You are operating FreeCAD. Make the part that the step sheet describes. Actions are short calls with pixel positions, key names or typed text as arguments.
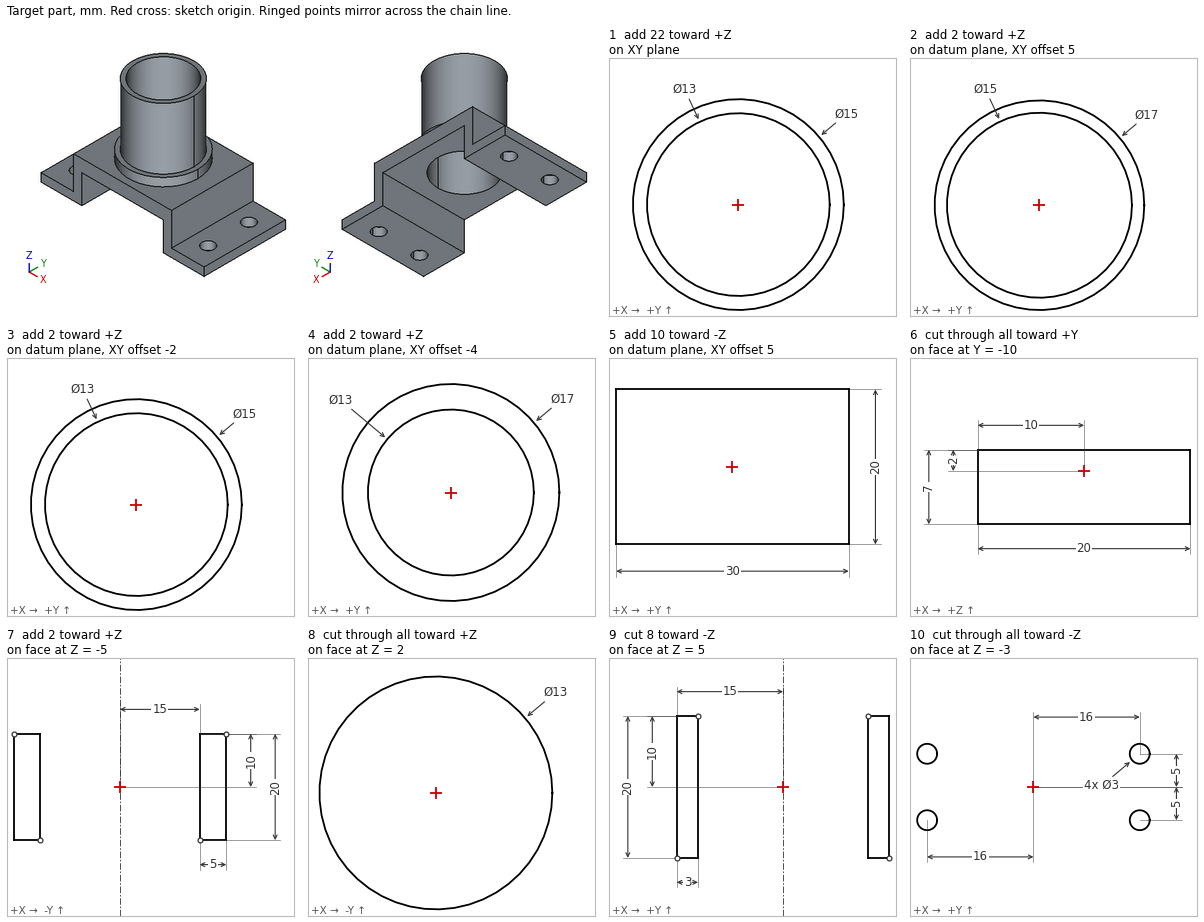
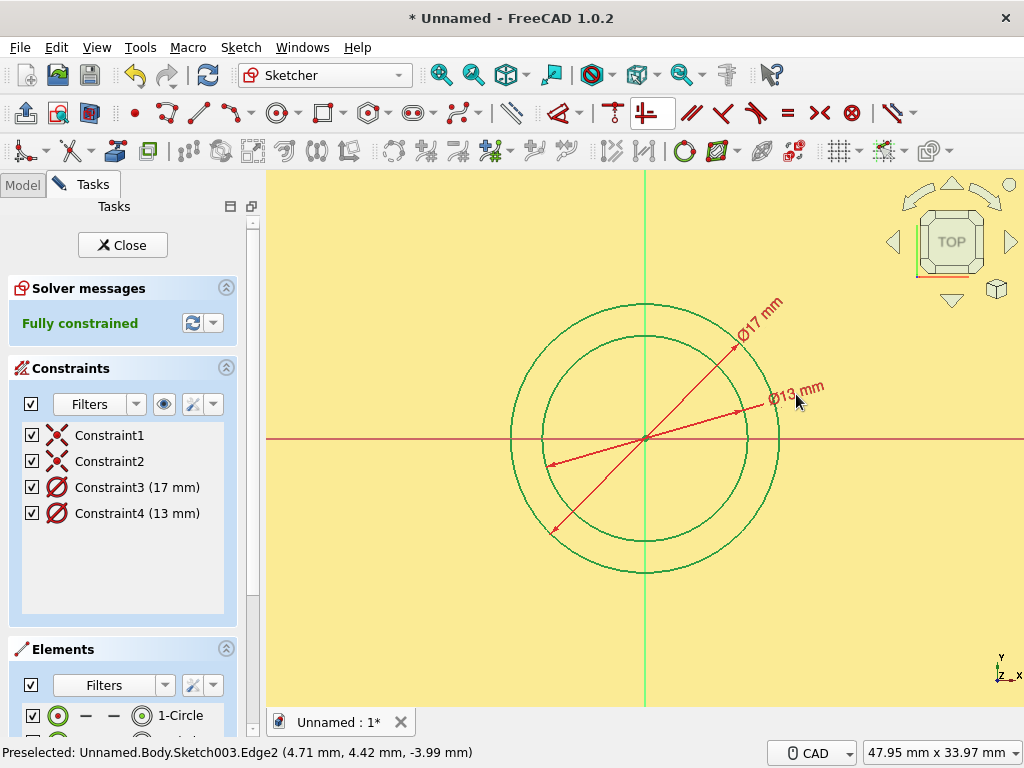
click(123, 245)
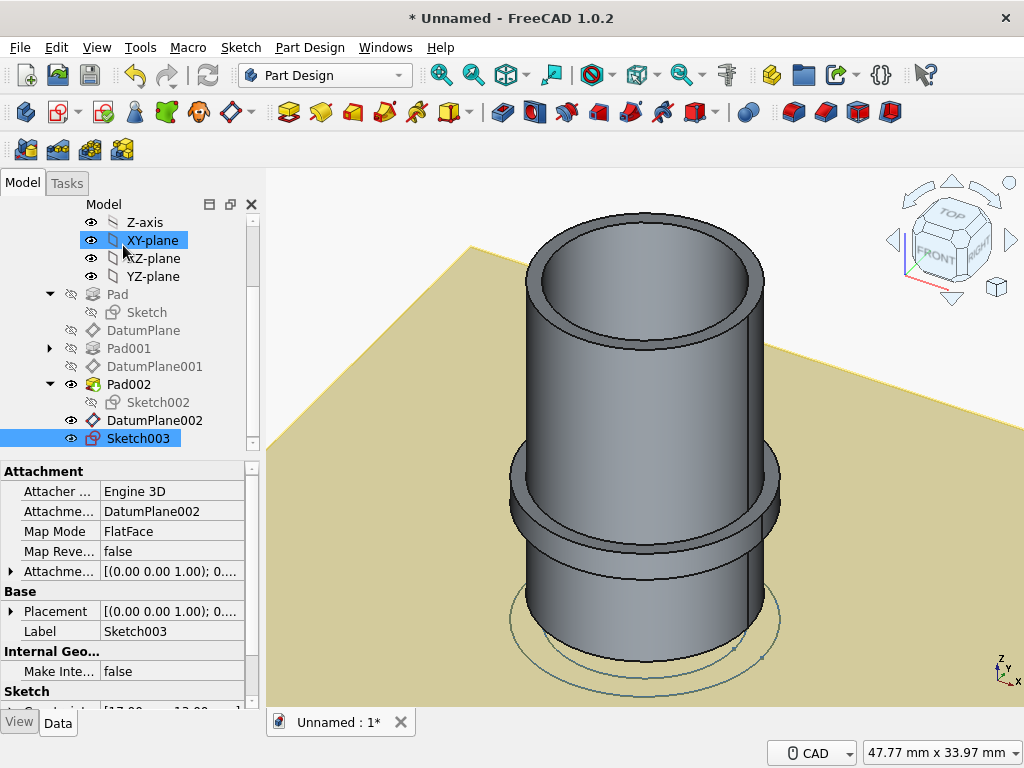
click(290, 112)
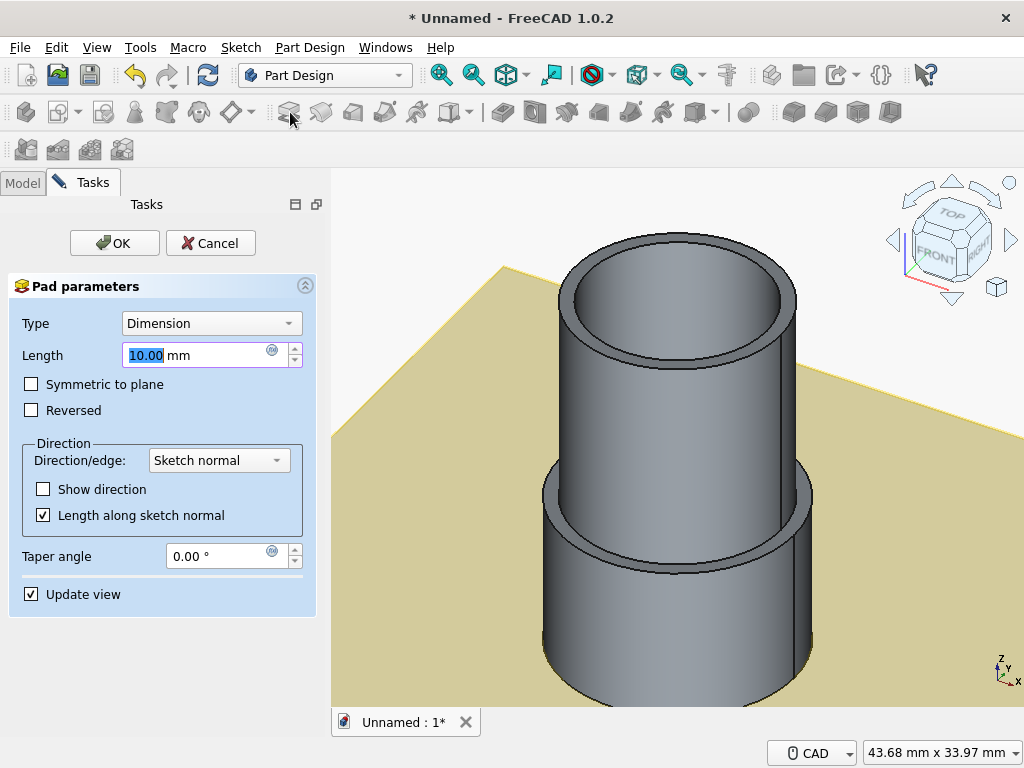
text(2)
key(Tab)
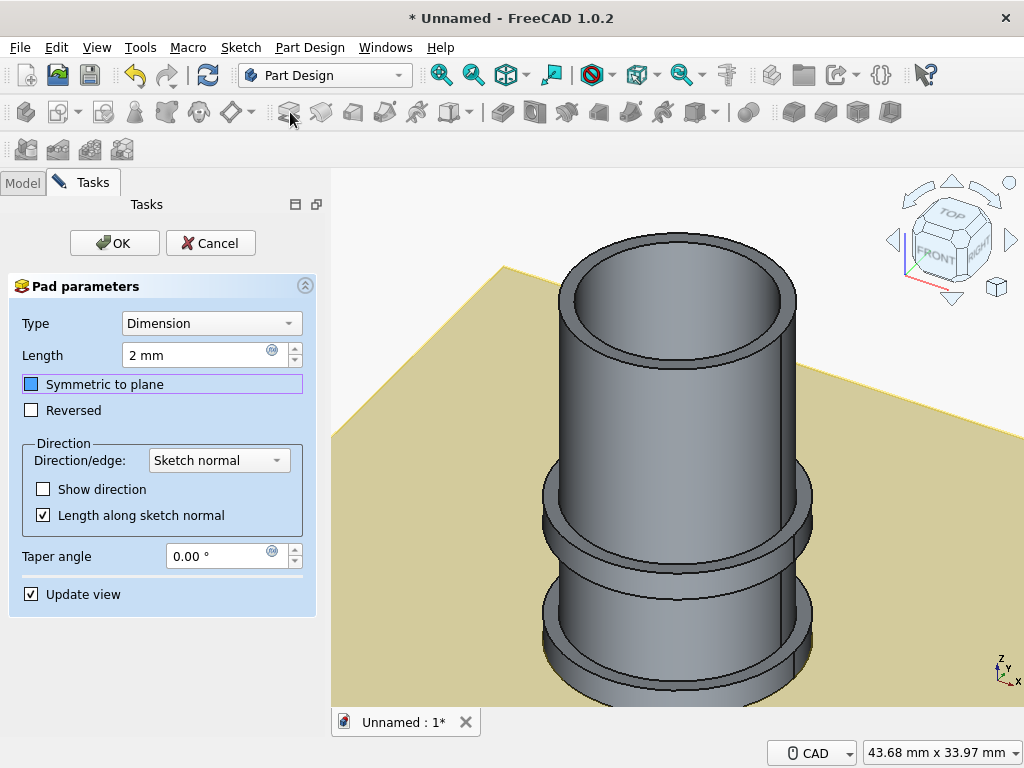
click(115, 243)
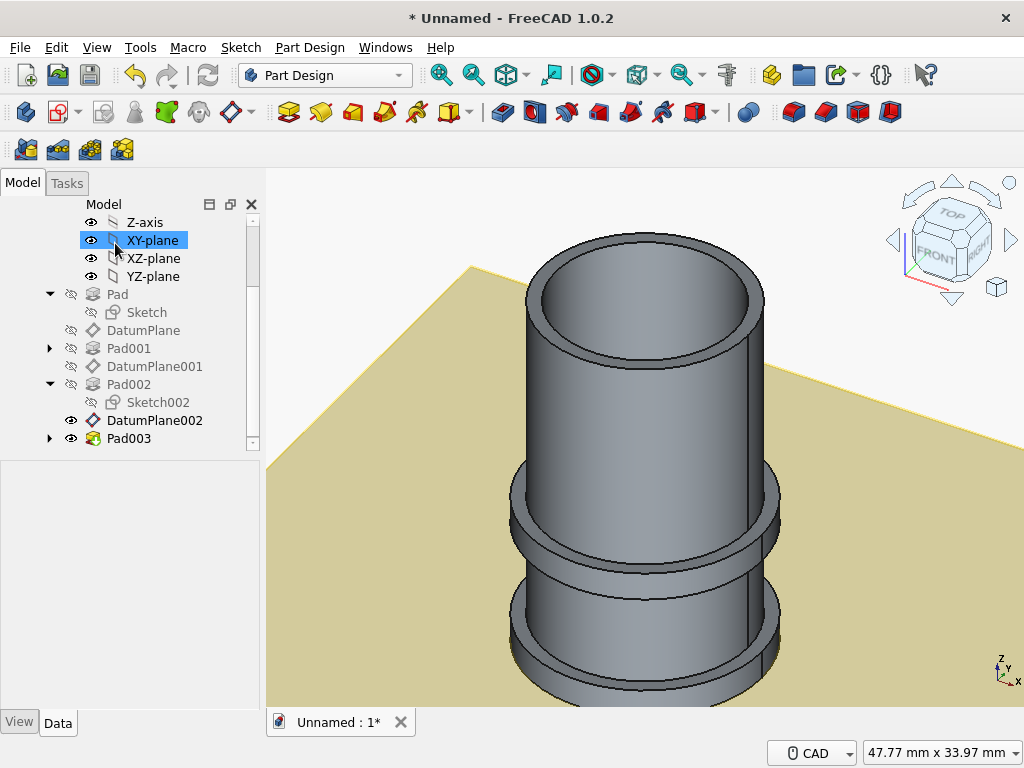
click(116, 420)
key(space)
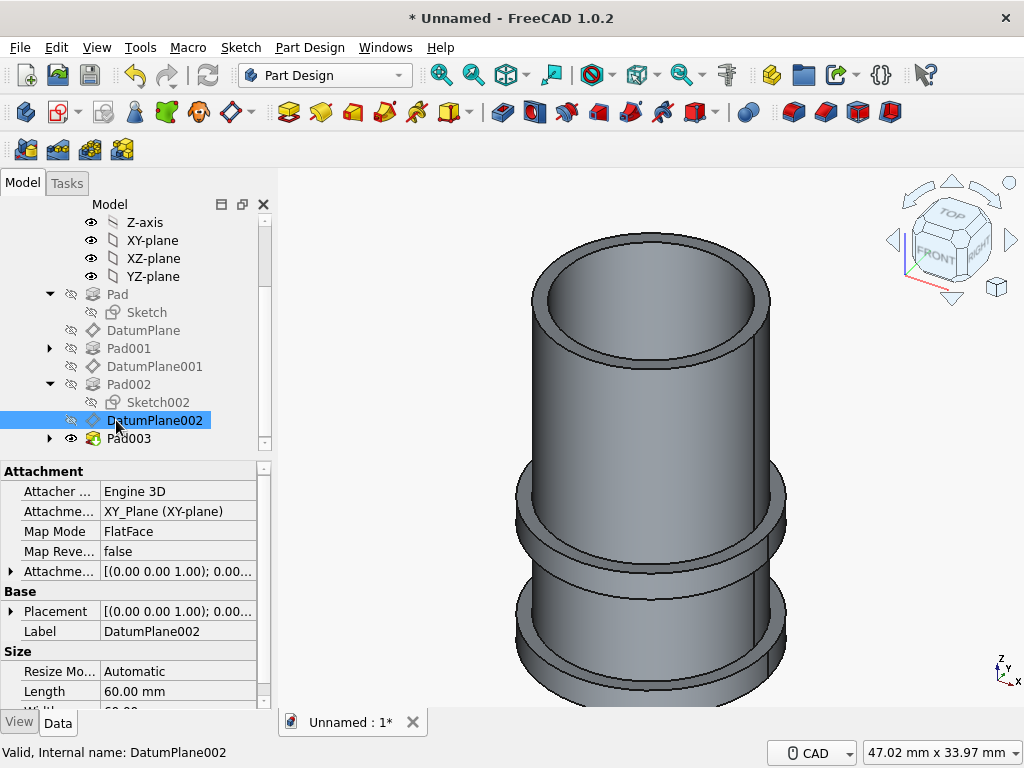
click(442, 76)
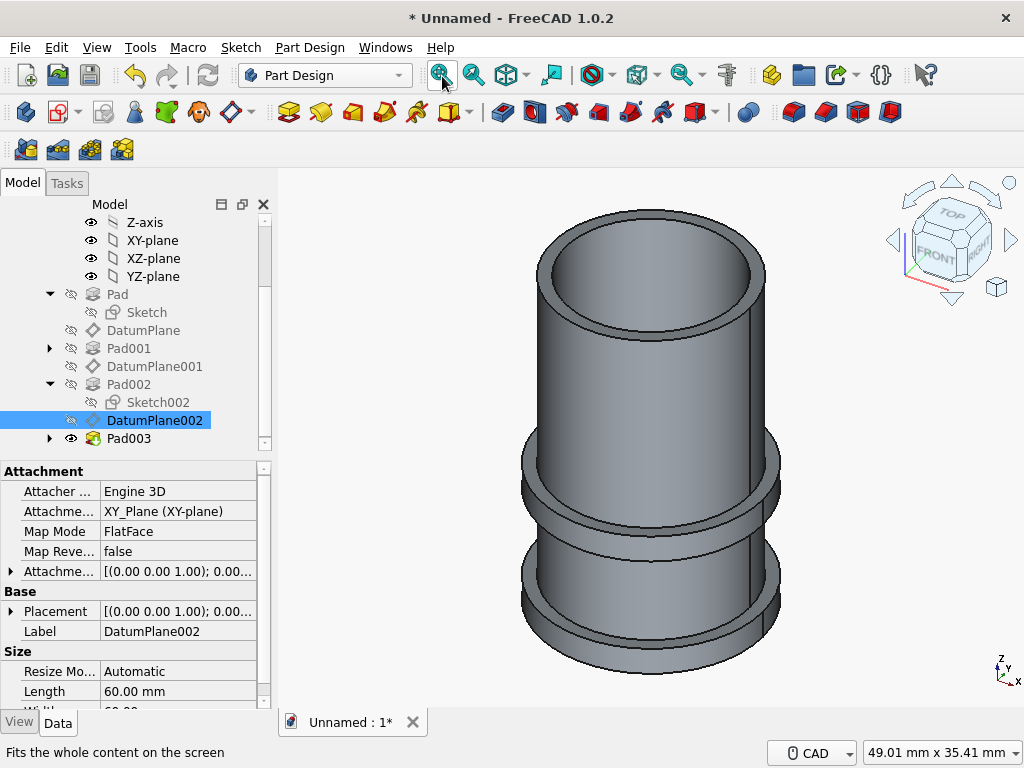
scroll(160, 326, down, 3)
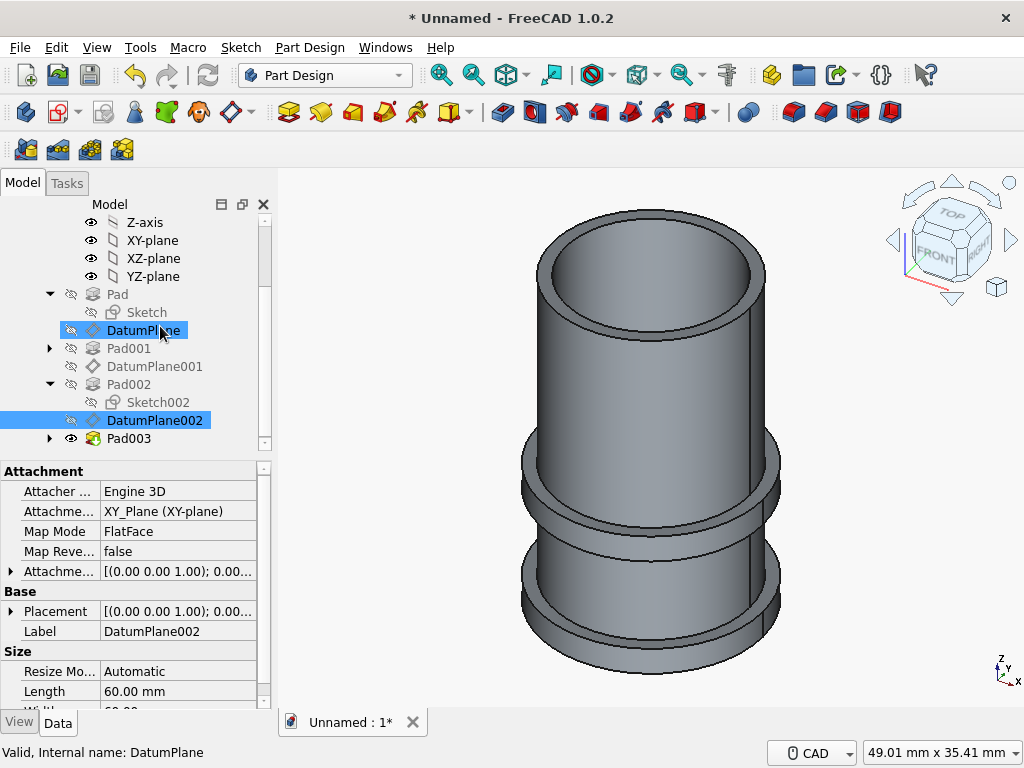
scroll(160, 326, up, 15)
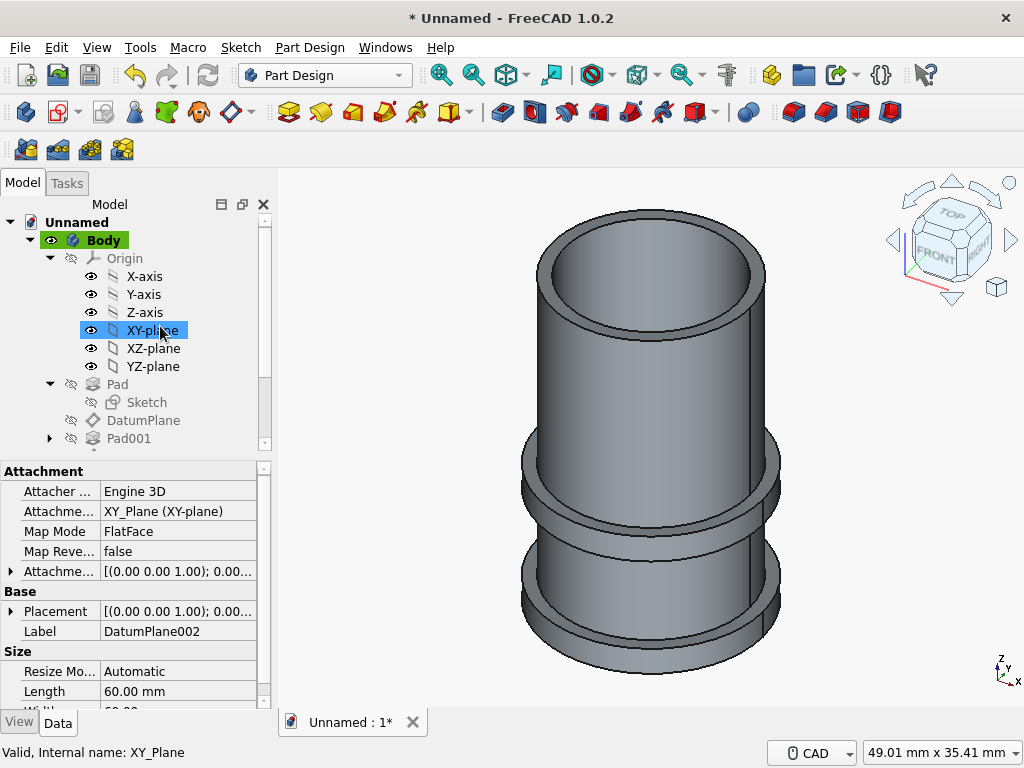
click(136, 330)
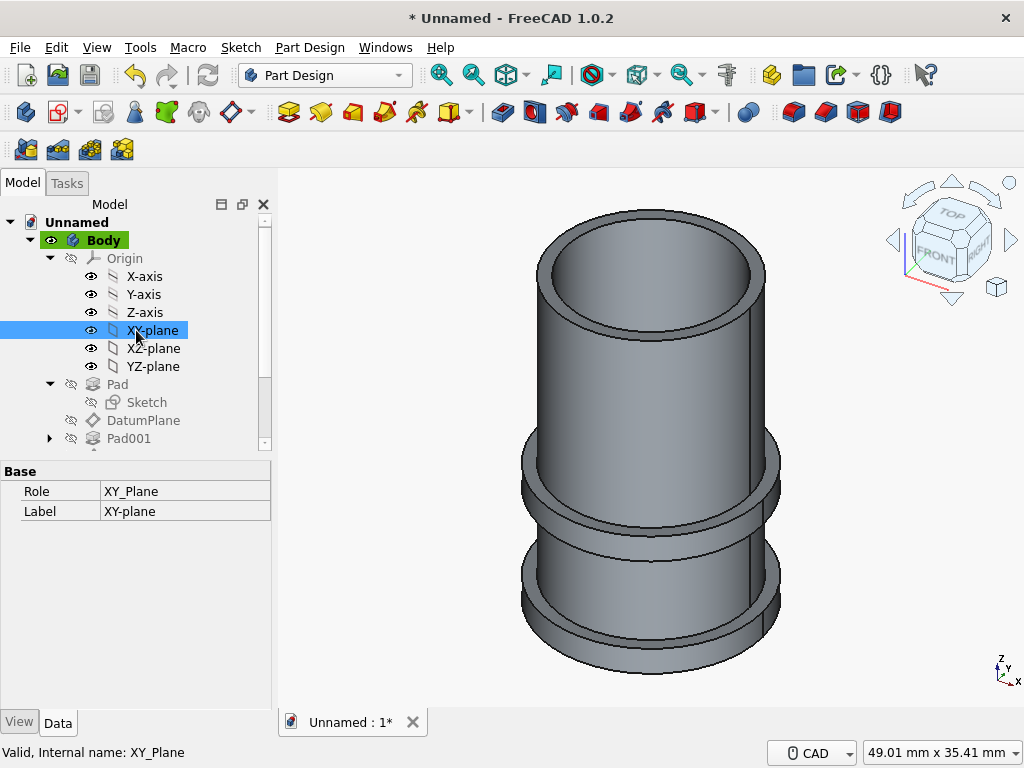
click(232, 112)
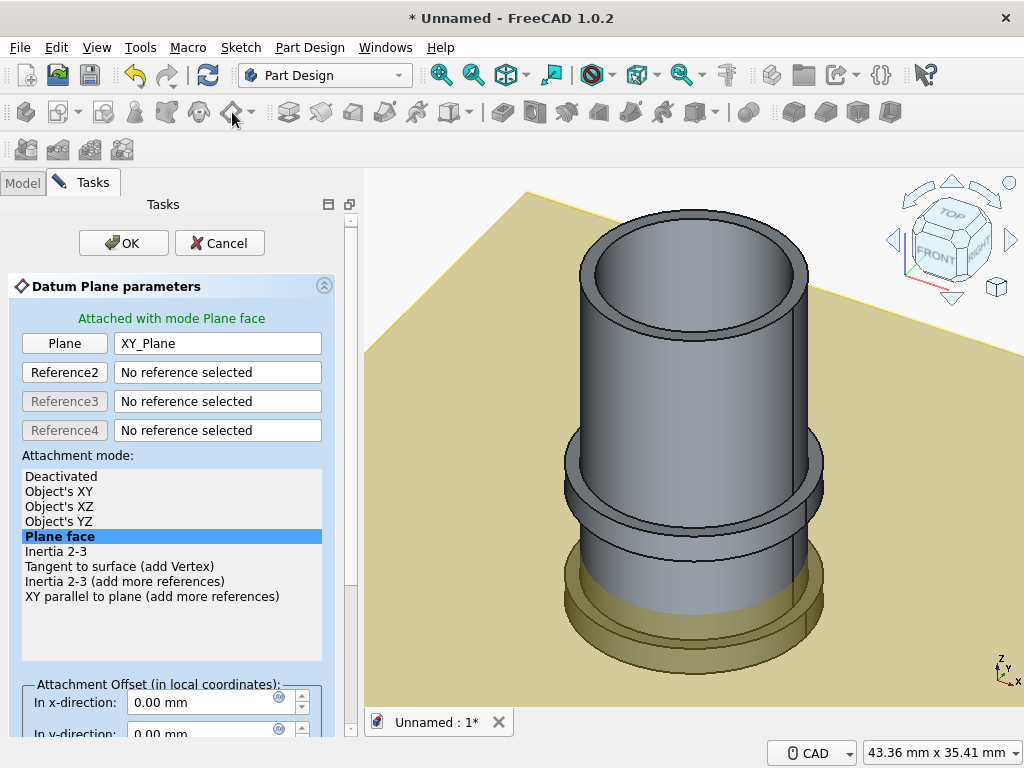
scroll(351, 475, down, 2)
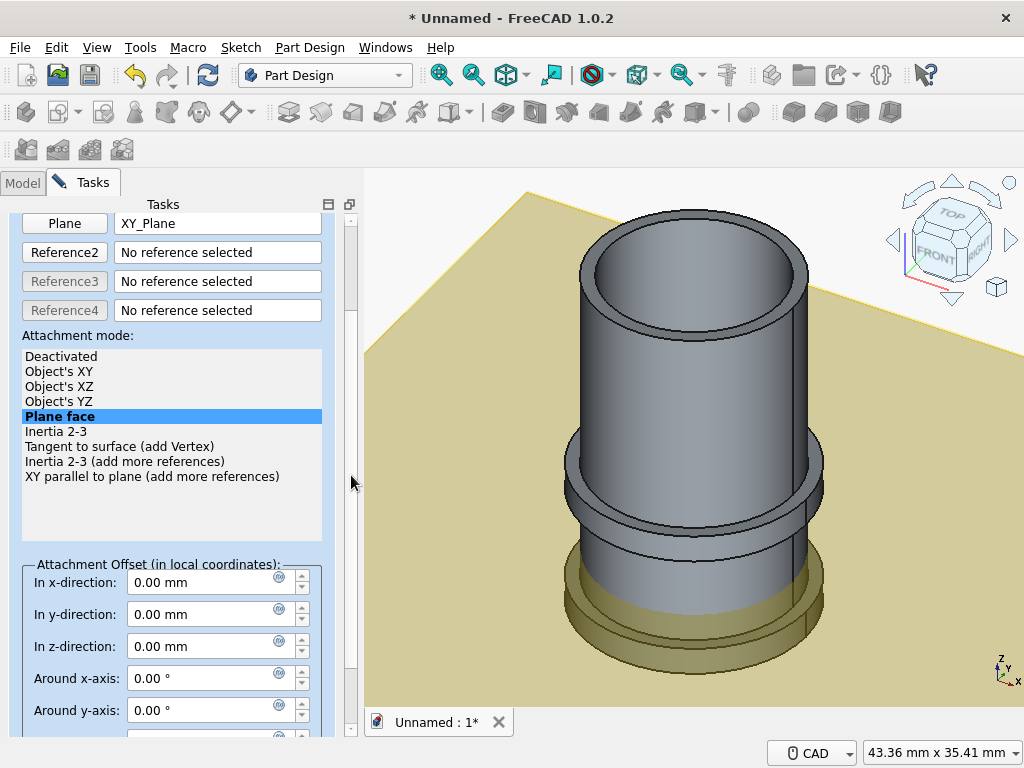
triple_click(210, 646)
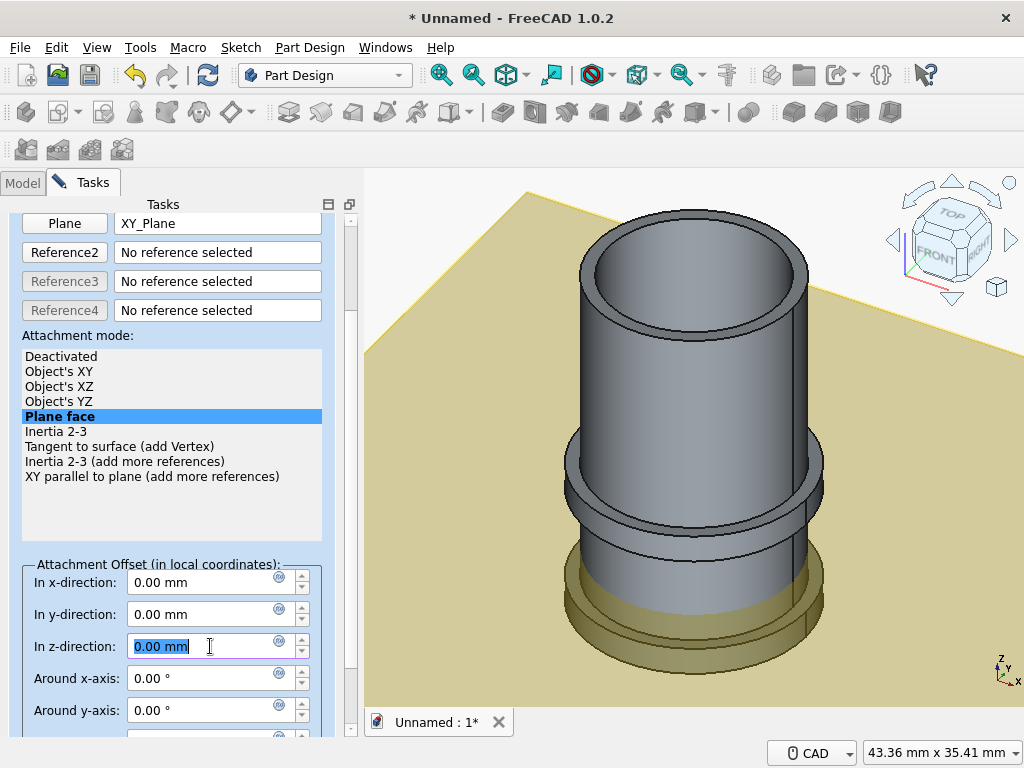
text(5)
key(Tab)